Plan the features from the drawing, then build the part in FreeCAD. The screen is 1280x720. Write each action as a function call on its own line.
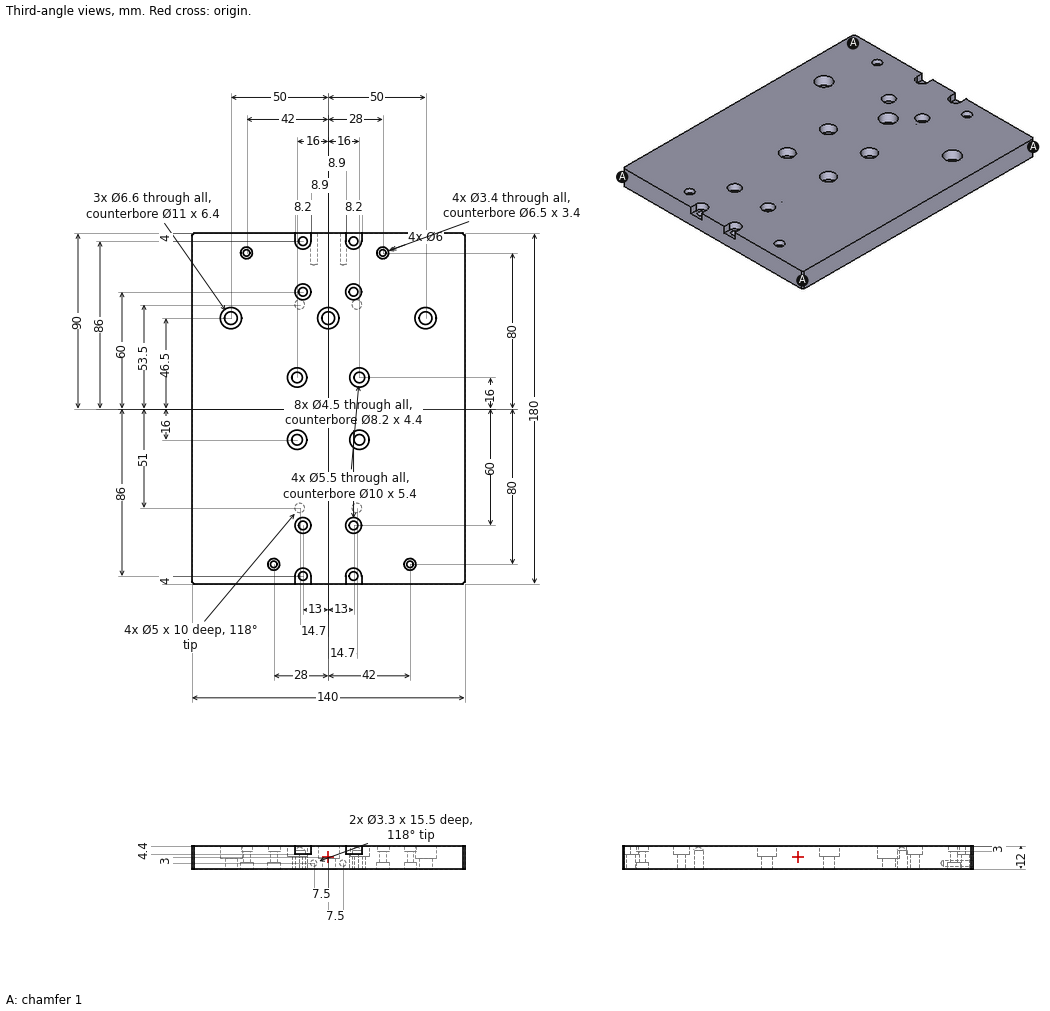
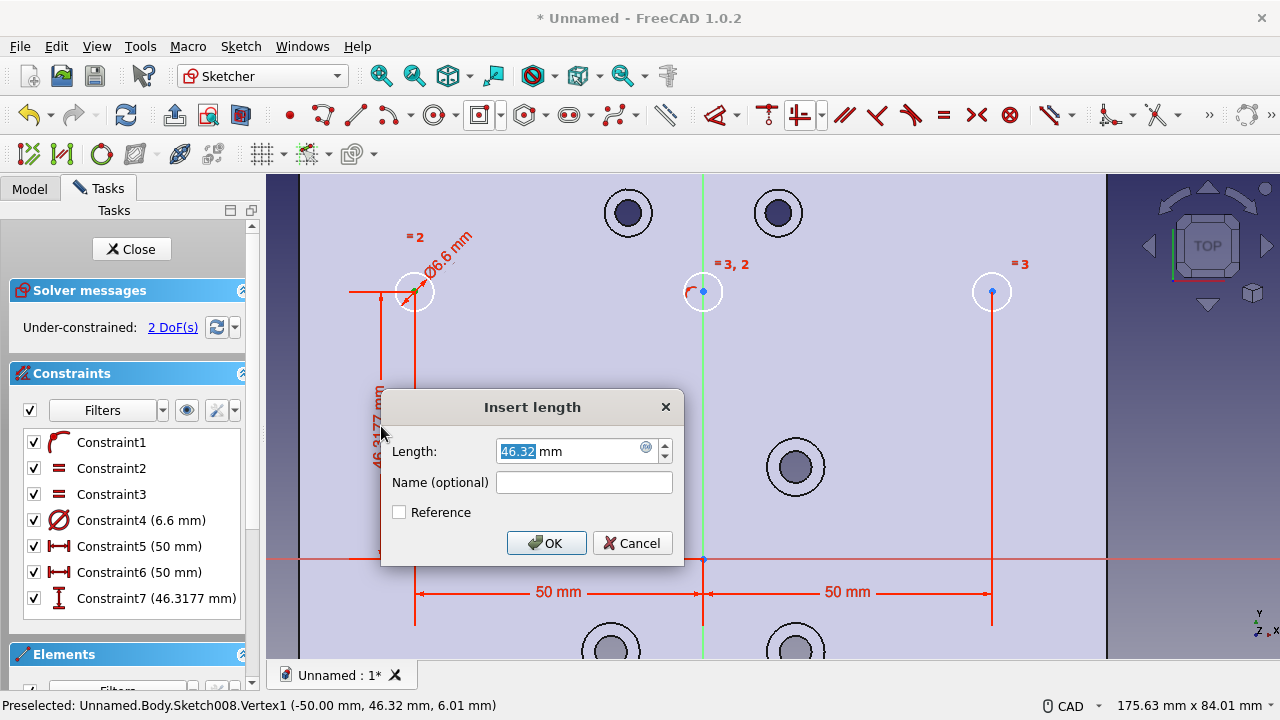
text(46.5)
key(Return)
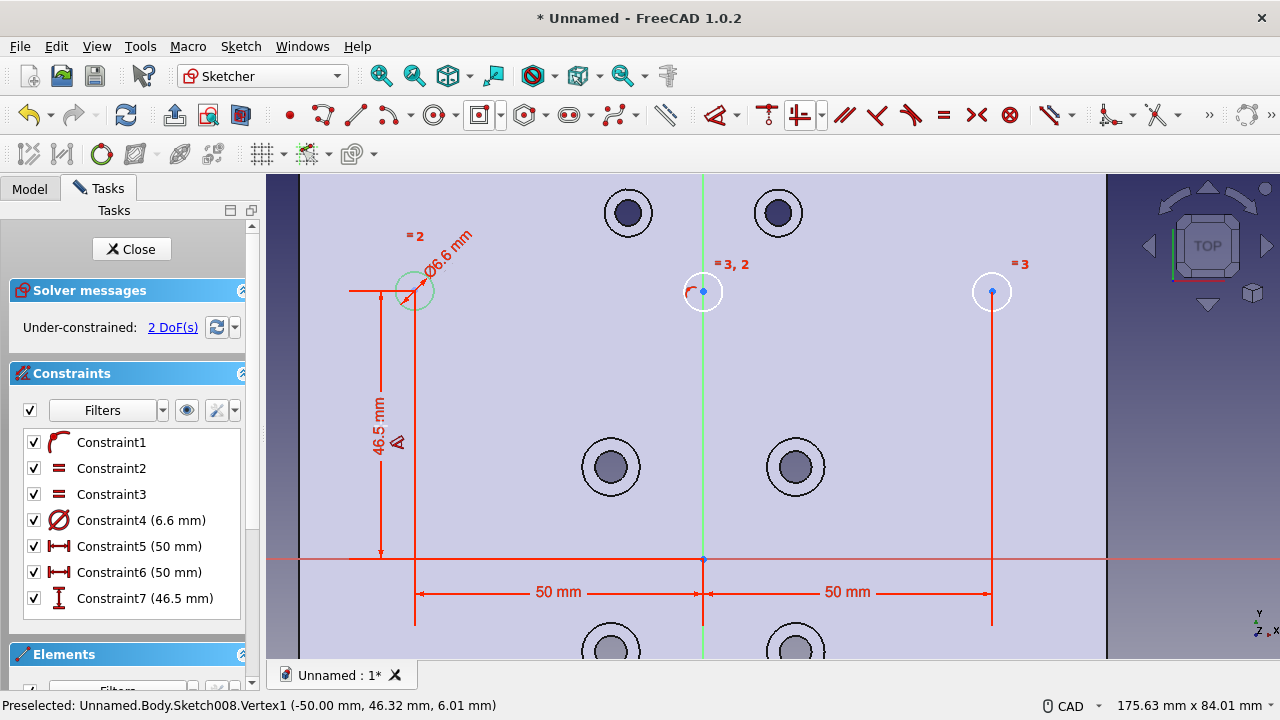
click(703, 292)
click(737, 426)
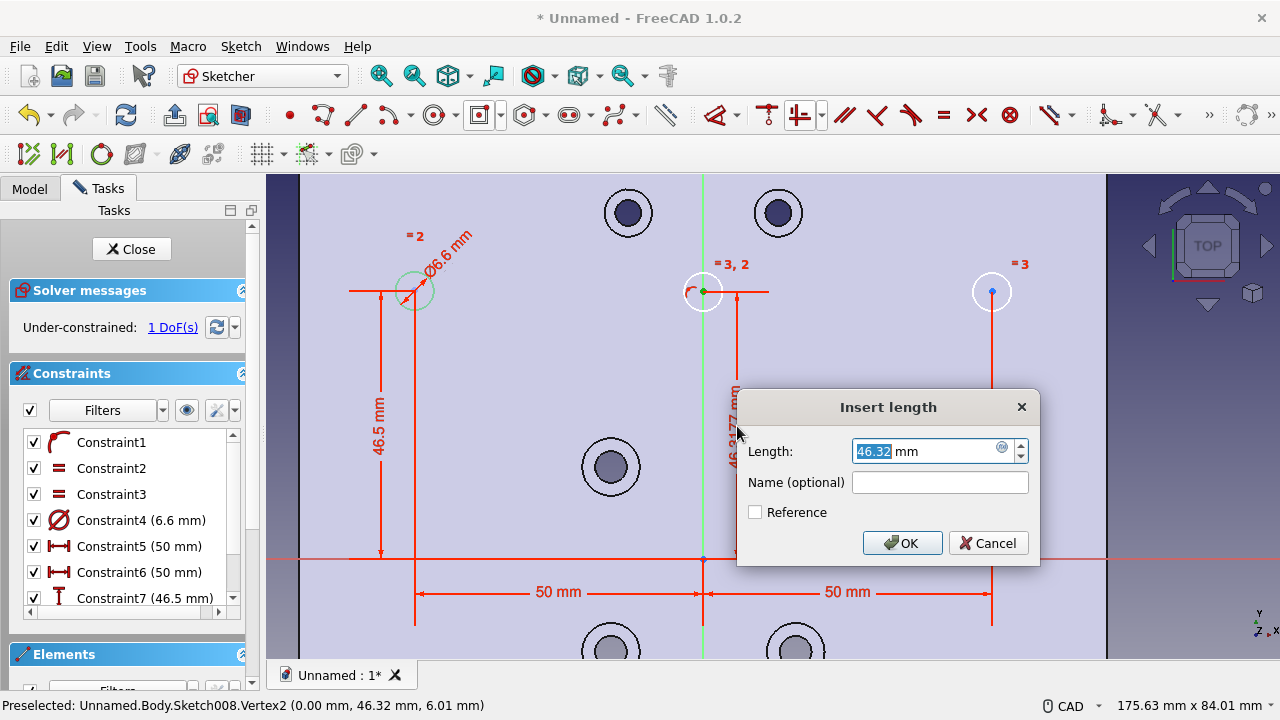
text(46.5)
key(Return)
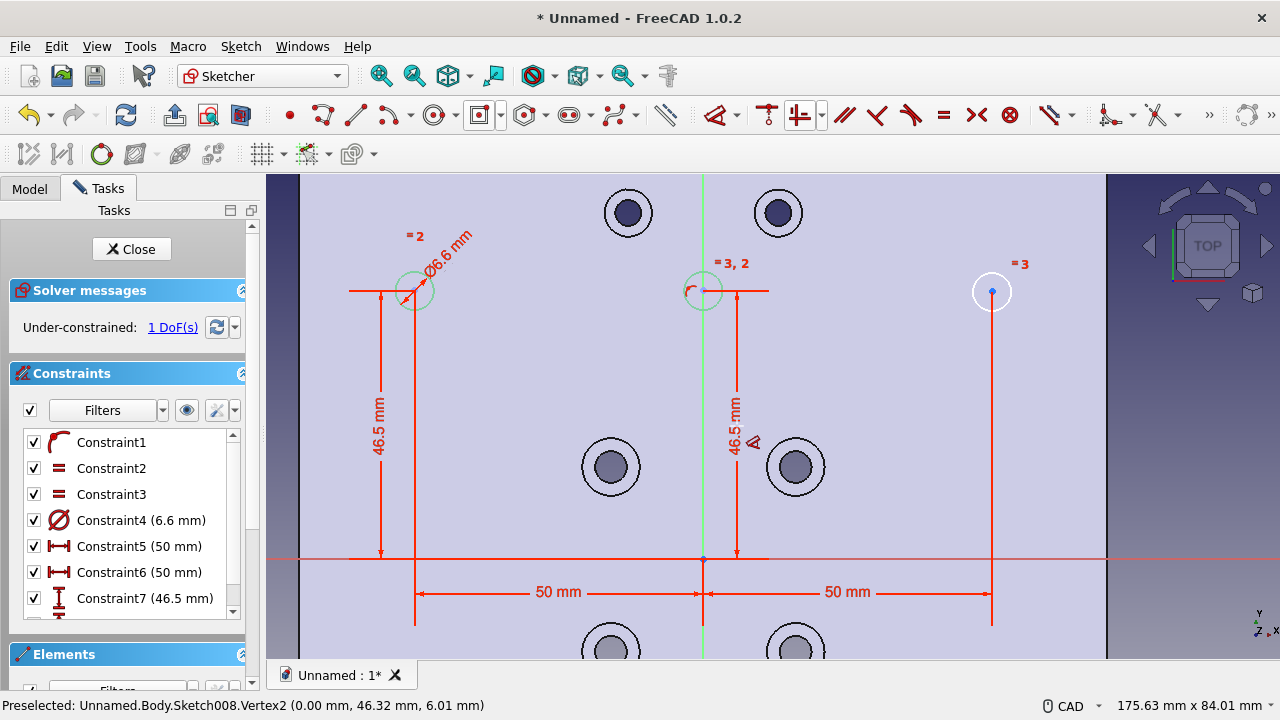
click(992, 292)
click(1026, 426)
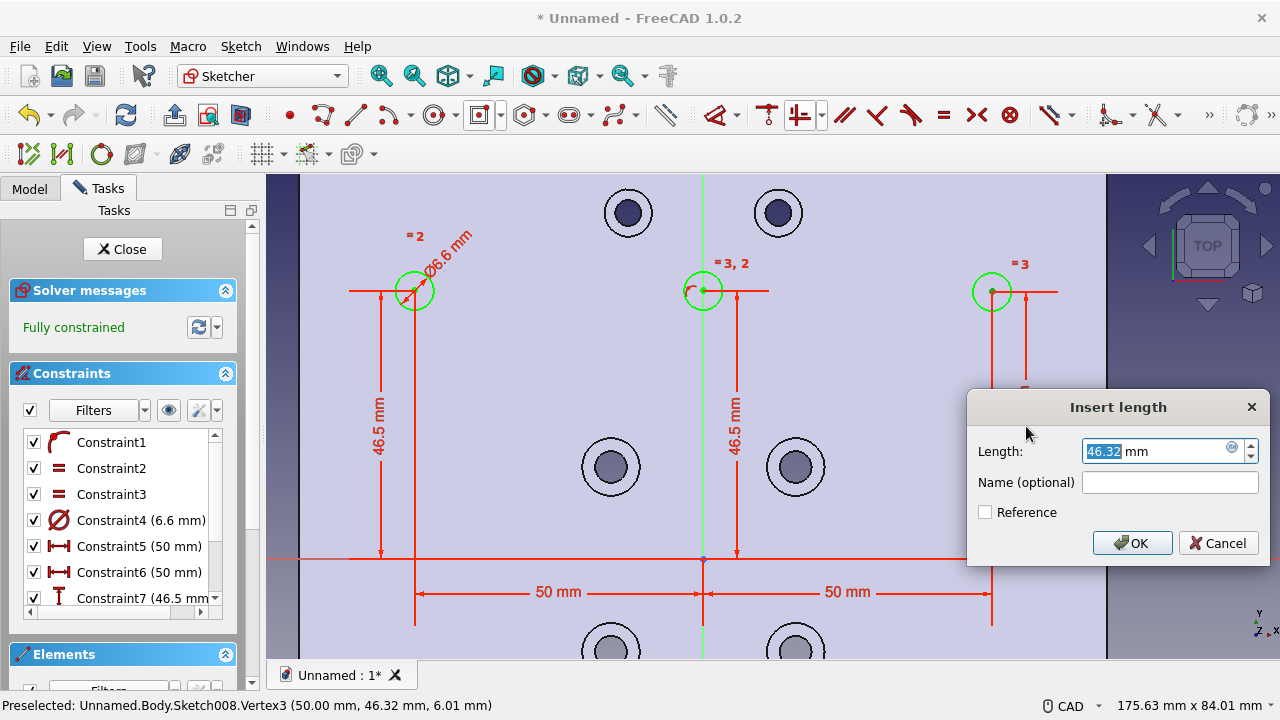
text(46.5)
key(Return)
key(Escape)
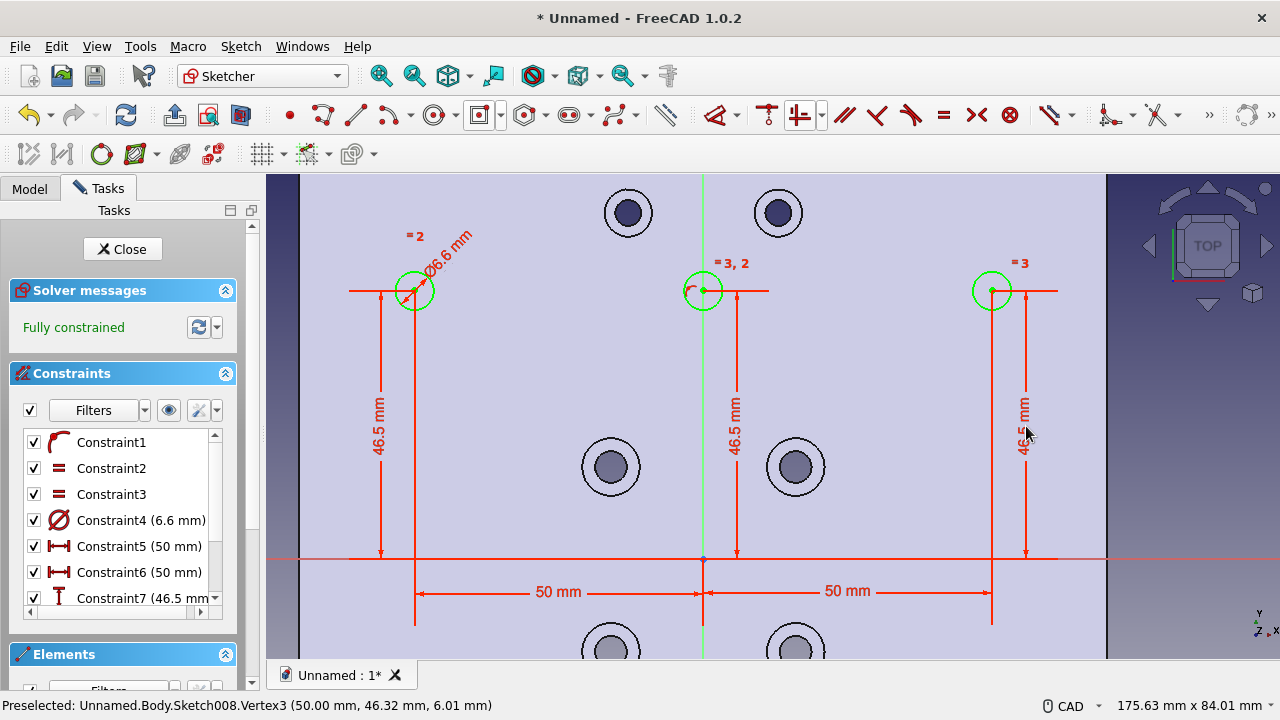
click(123, 249)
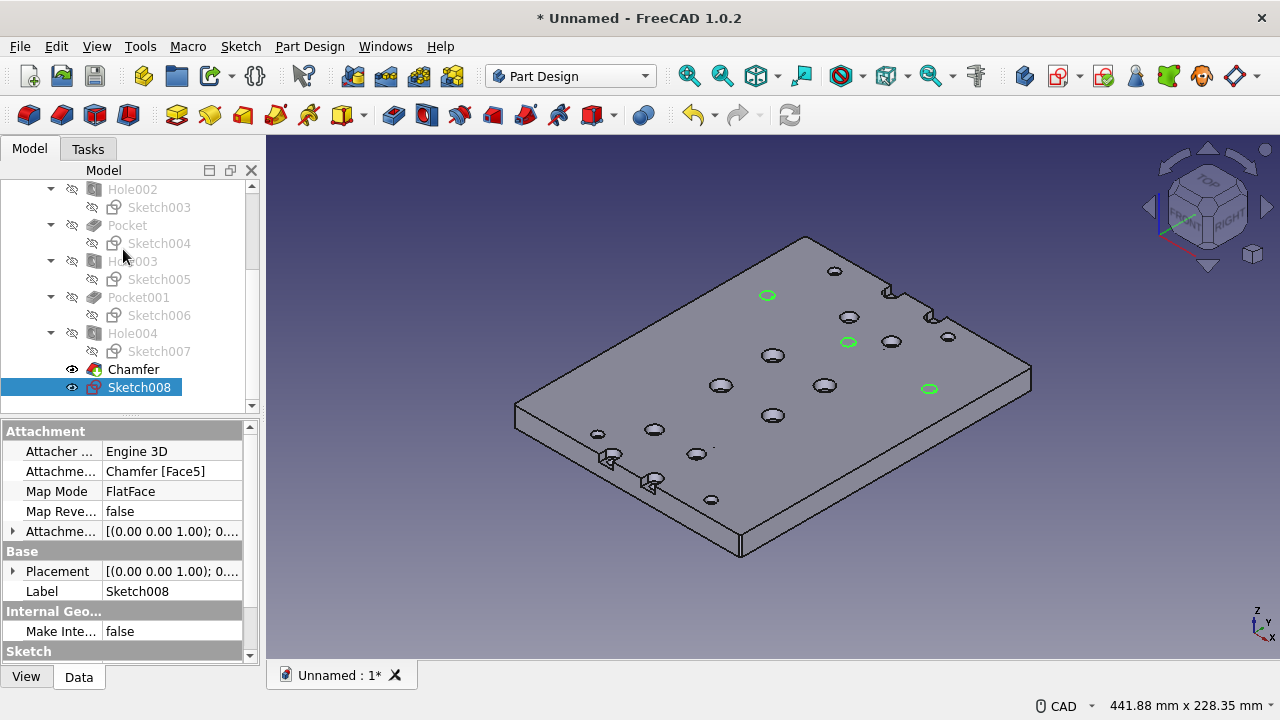
click(427, 116)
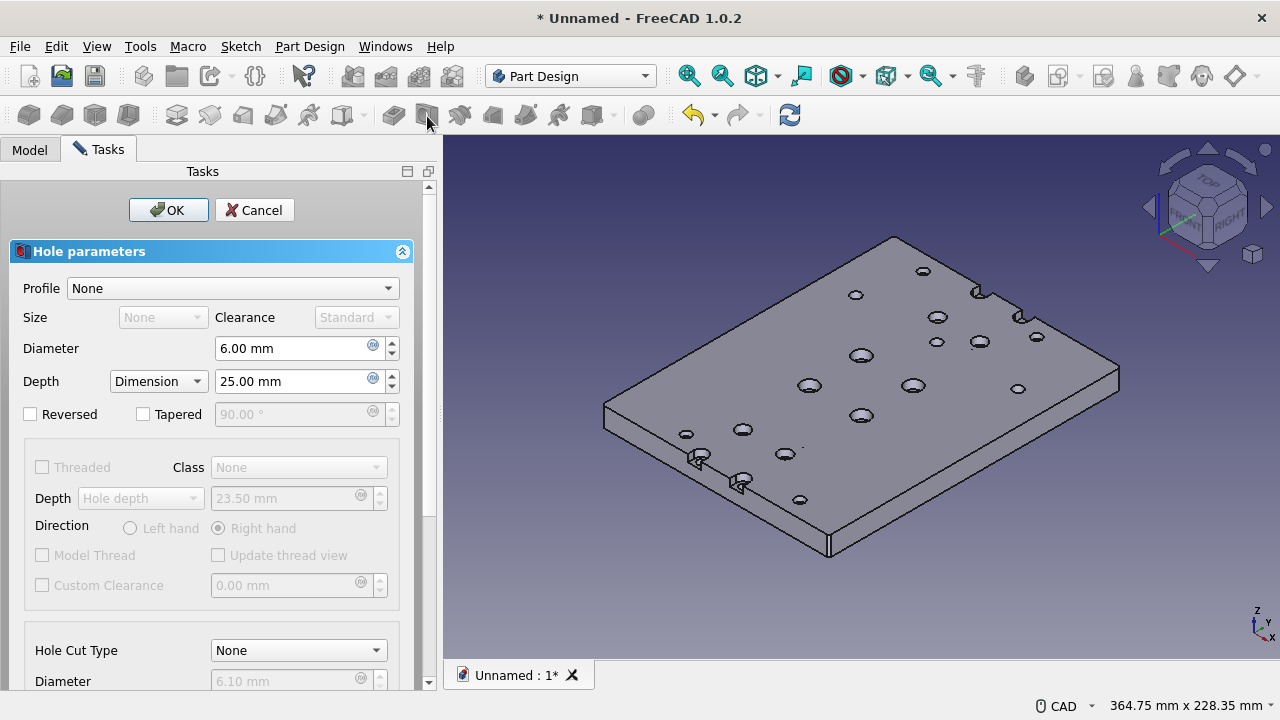
triple_click(300, 348)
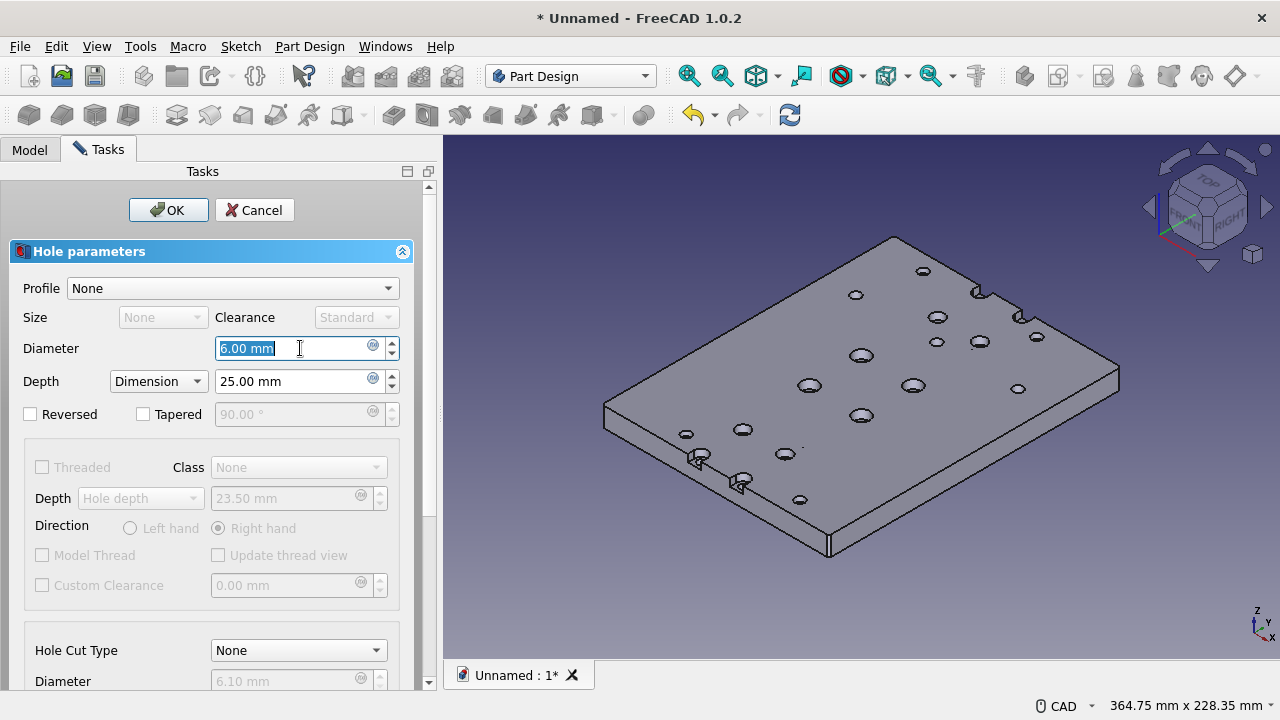
text(6.6)
key(Tab)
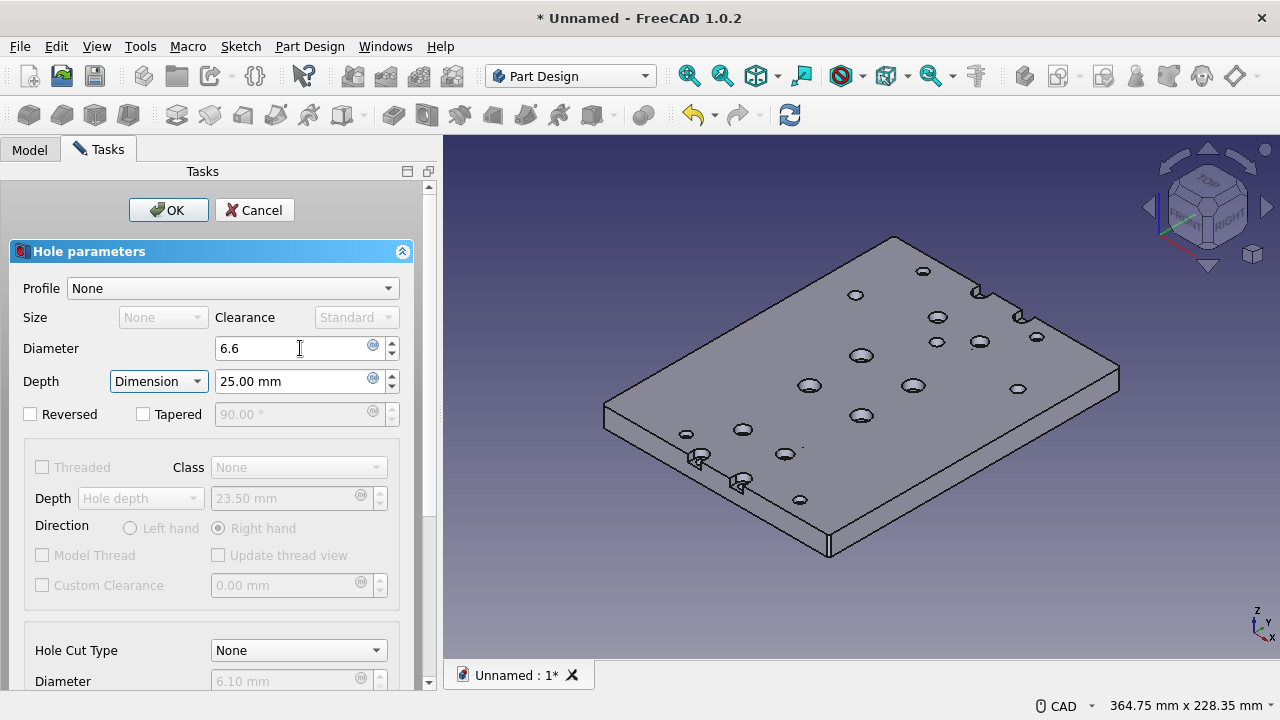
click(160, 382)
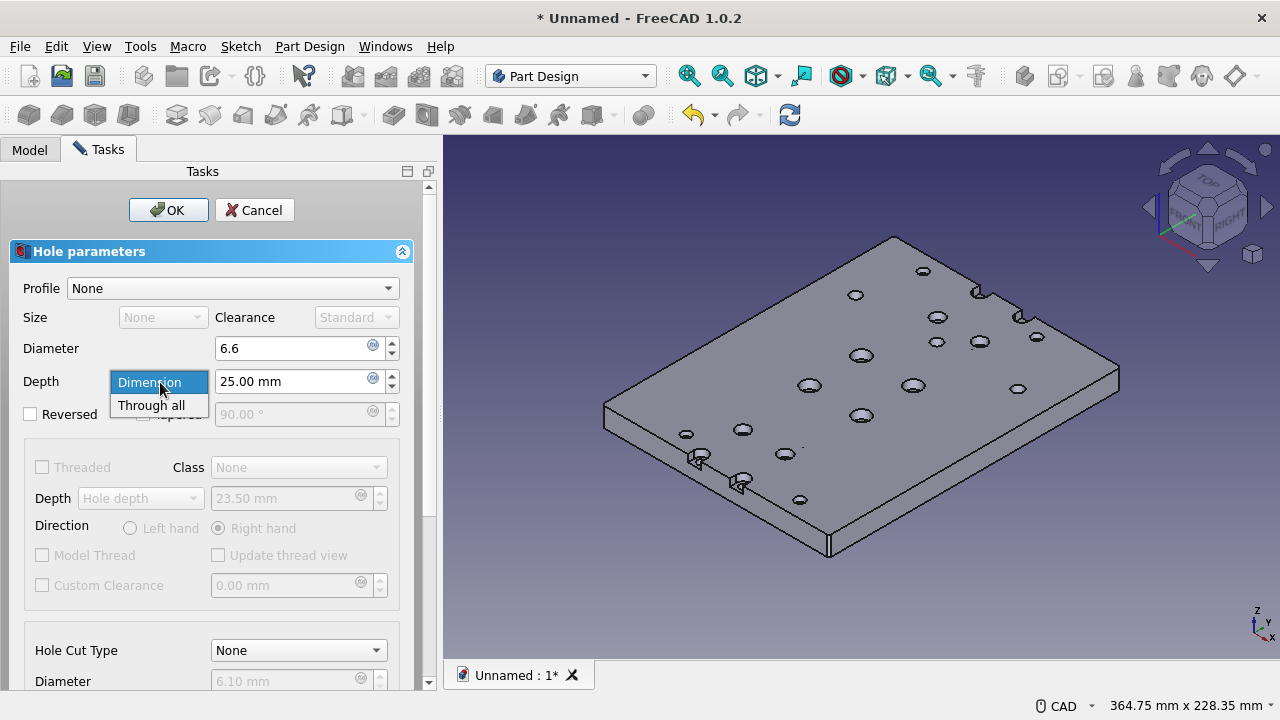
click(158, 406)